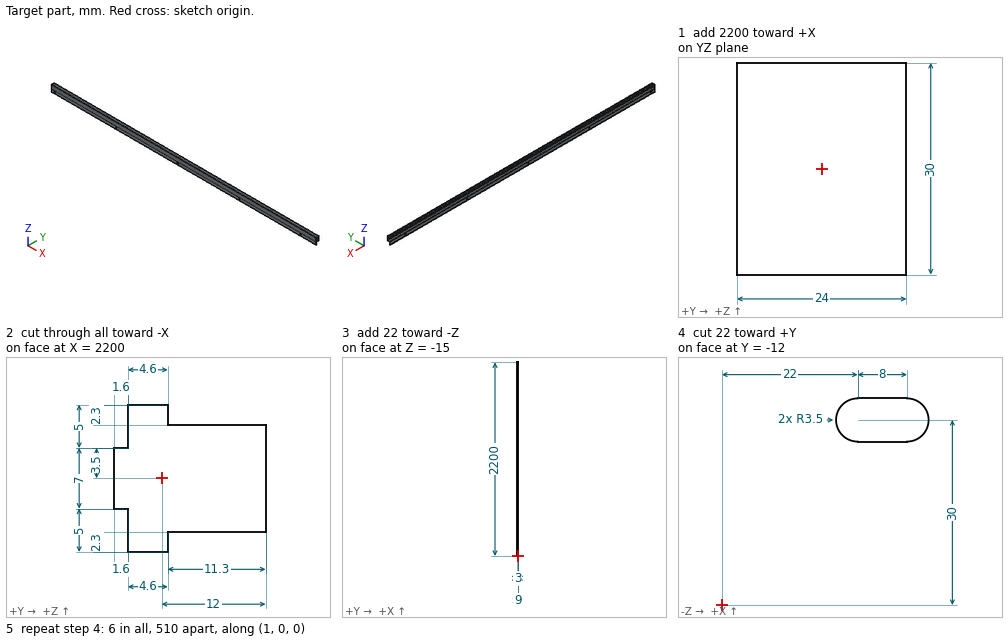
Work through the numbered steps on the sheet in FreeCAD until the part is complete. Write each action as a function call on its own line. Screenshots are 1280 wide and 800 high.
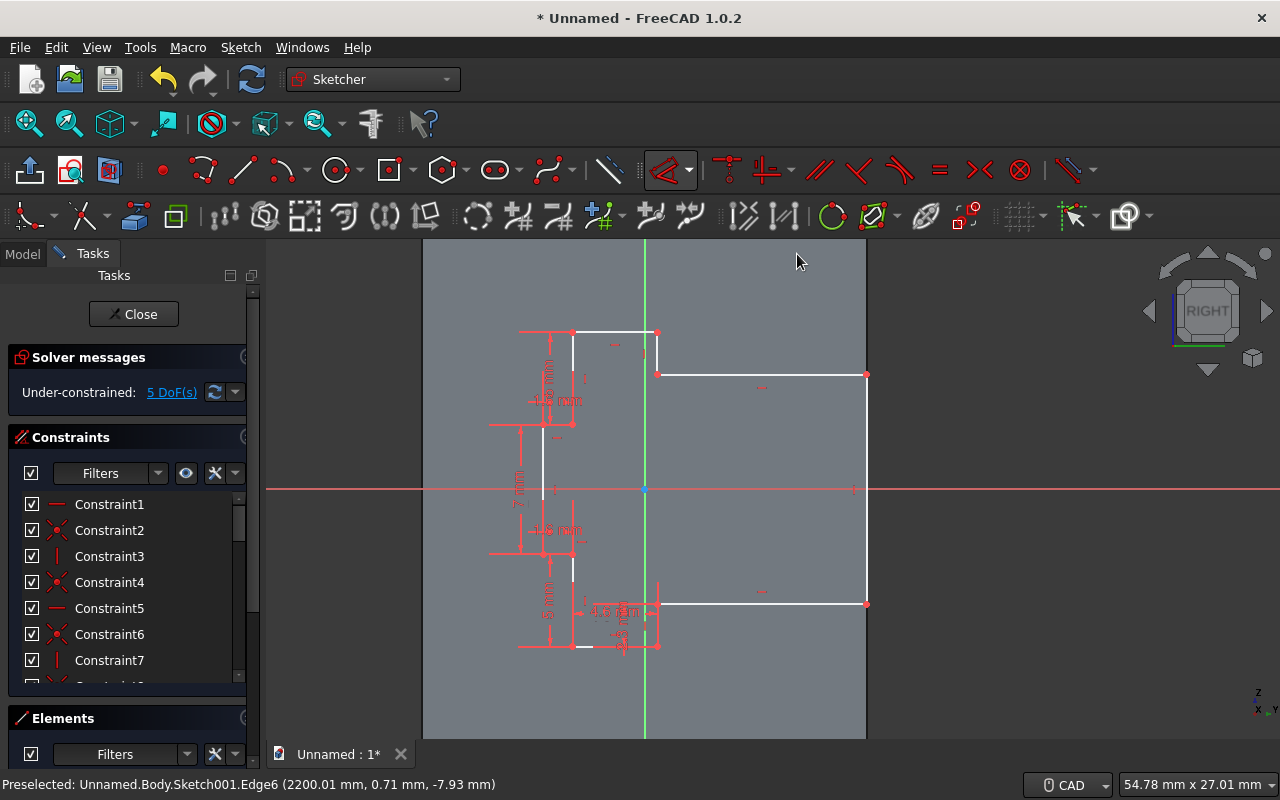
click(657, 362)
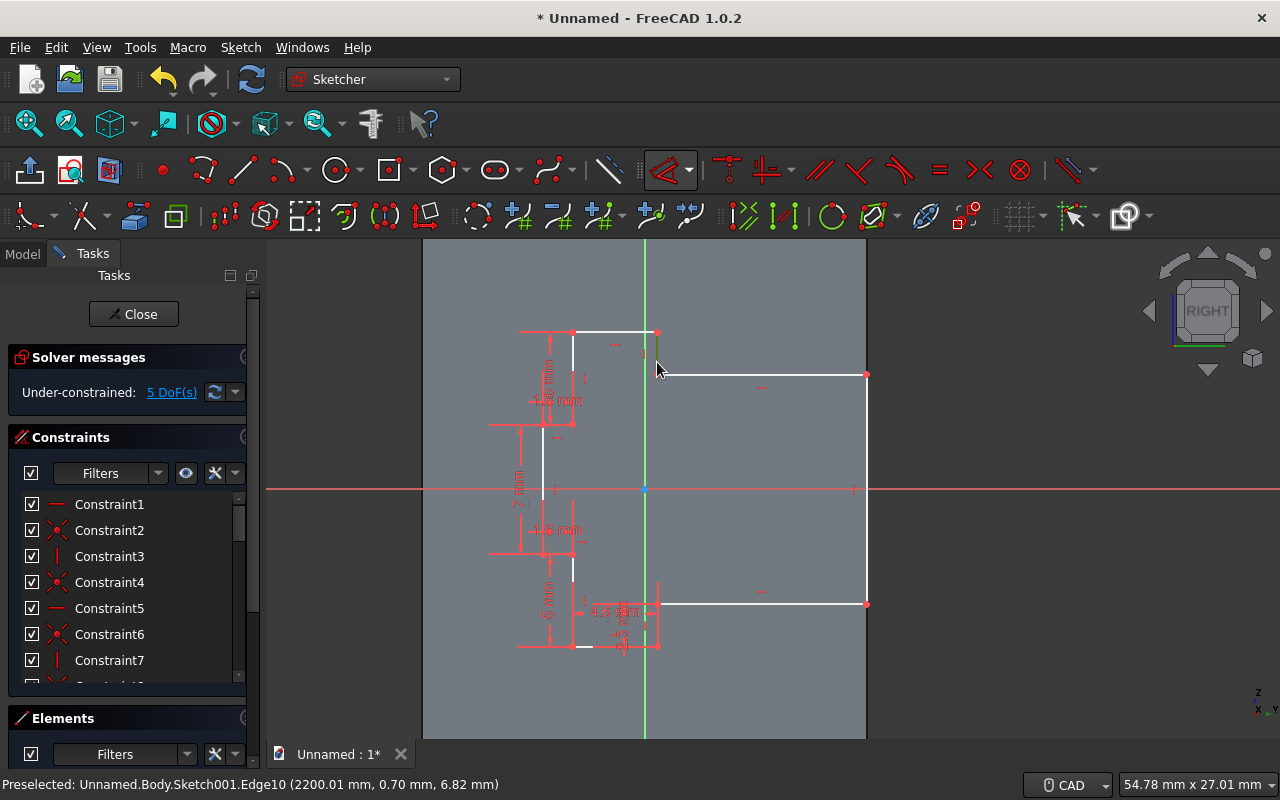
key(i)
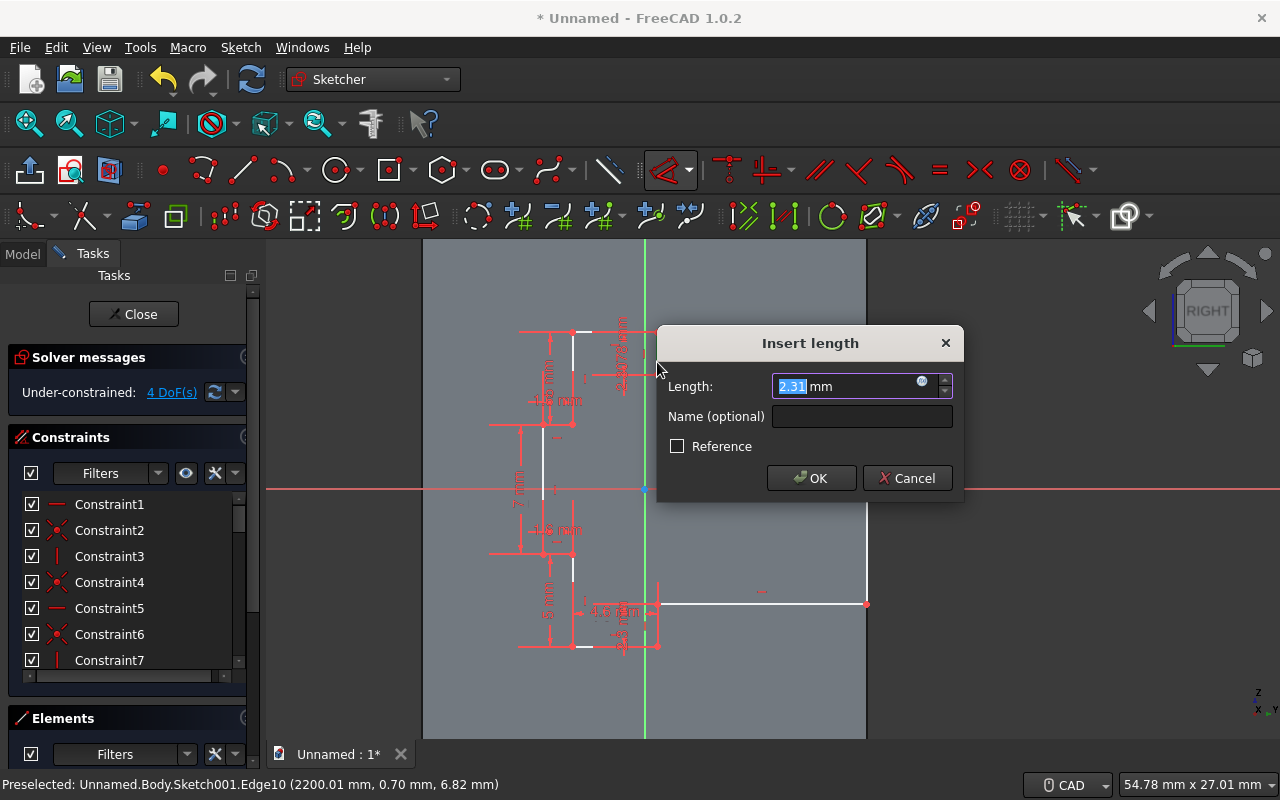
text(2.3)
key(Return)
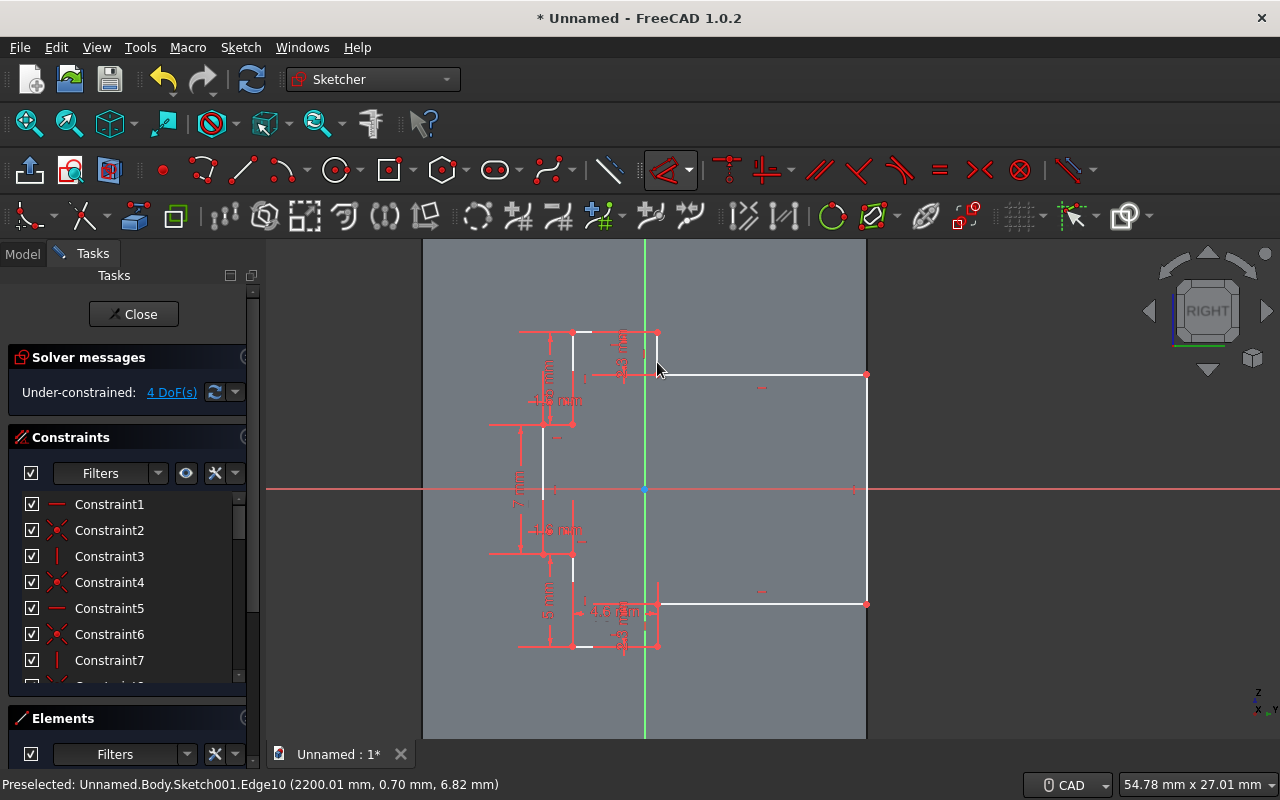
click(598, 332)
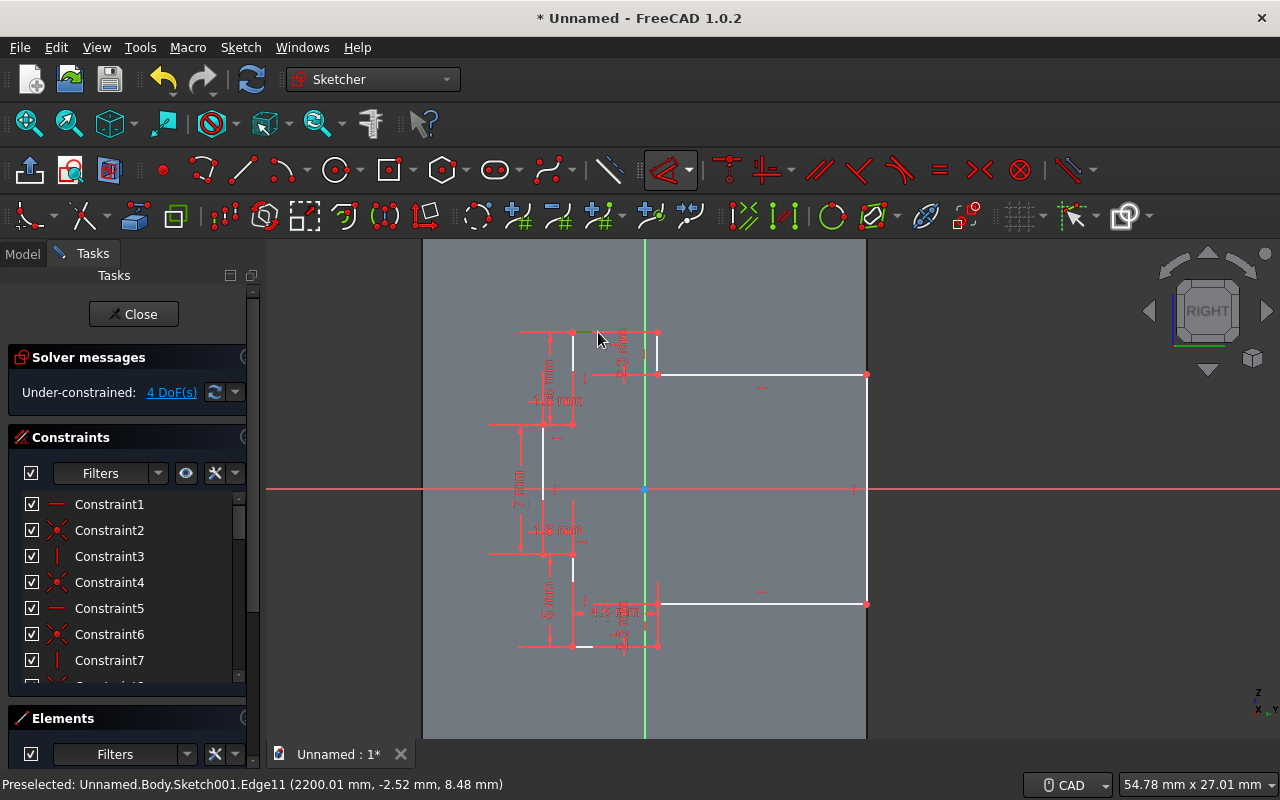
click(692, 170)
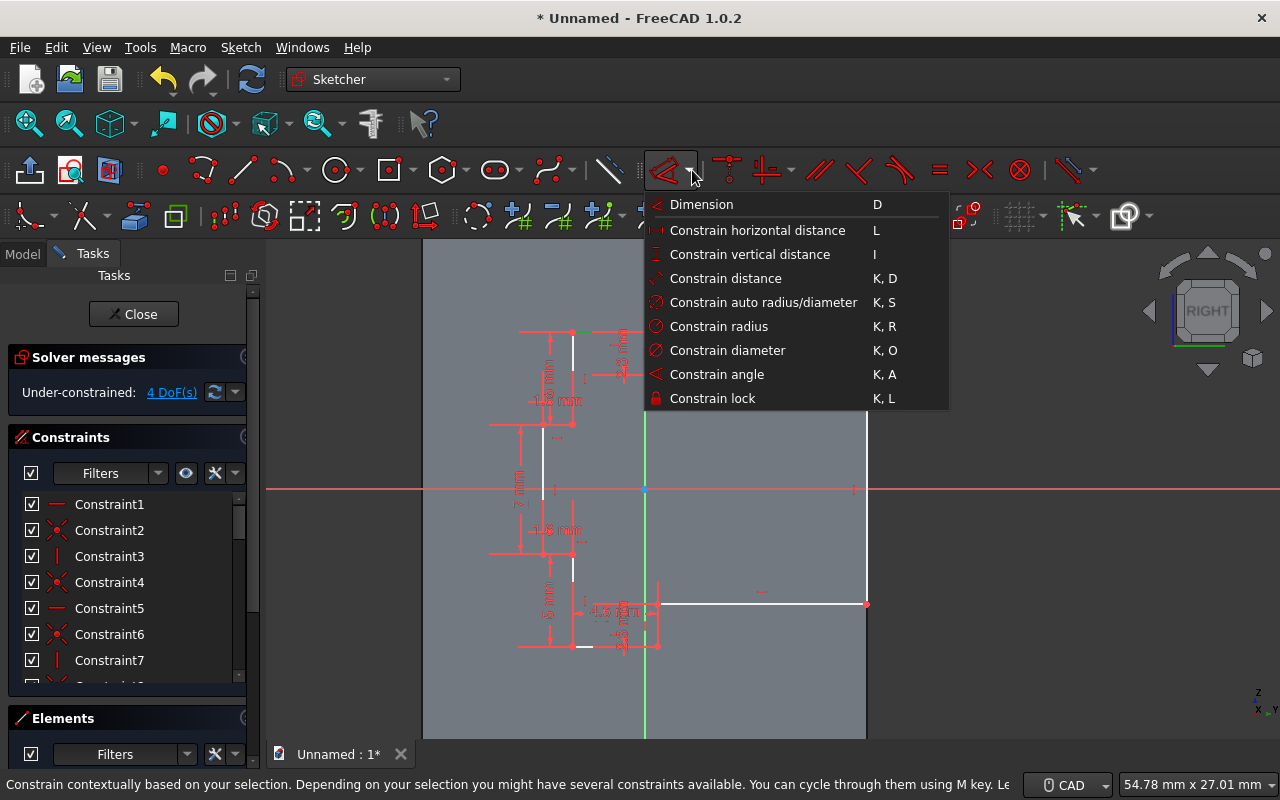
click(797, 230)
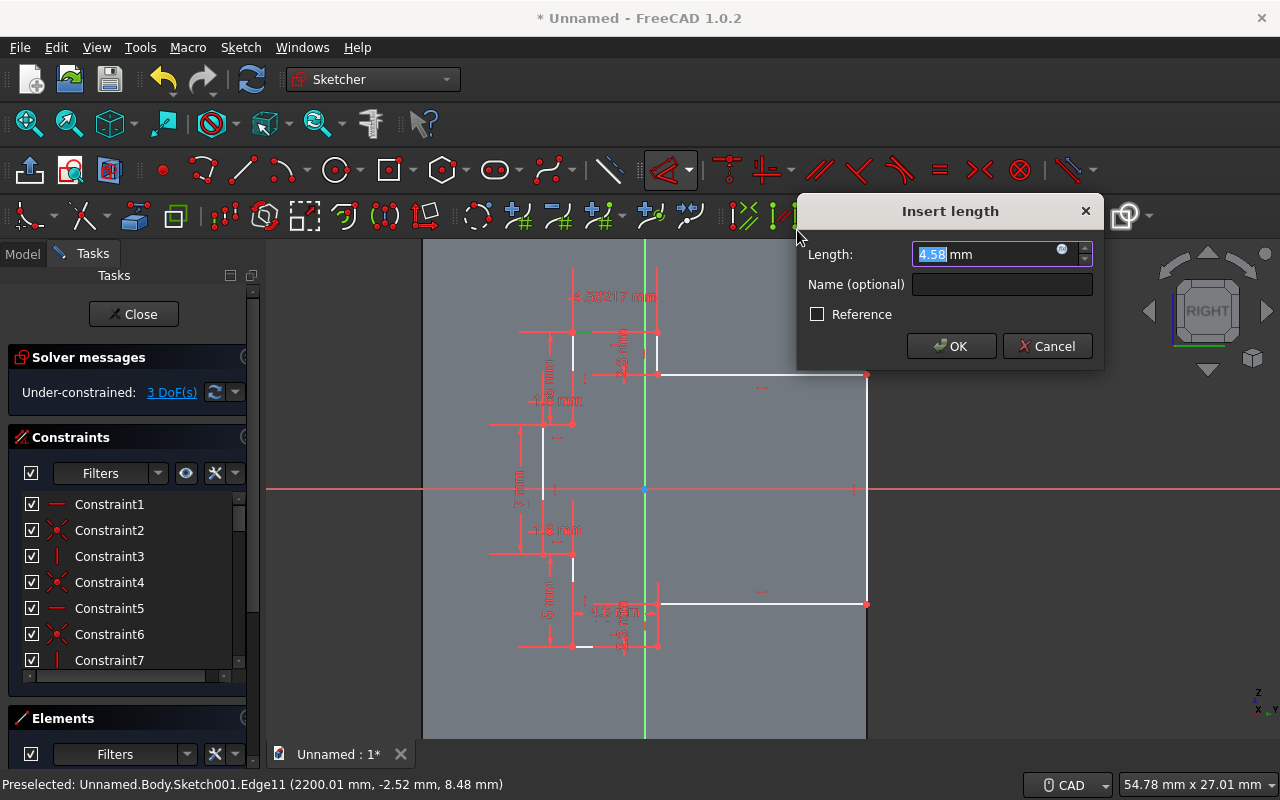
text(4.6)
key(Return)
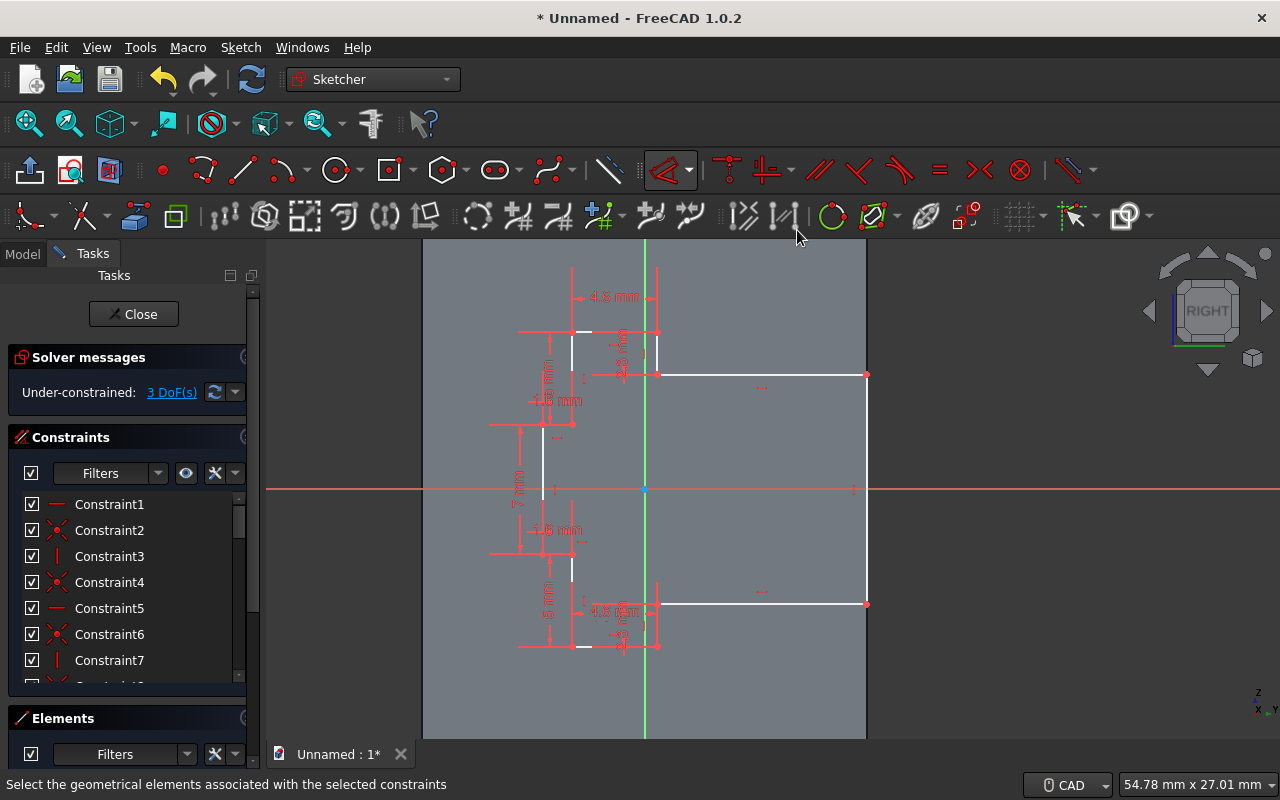
click(867, 604)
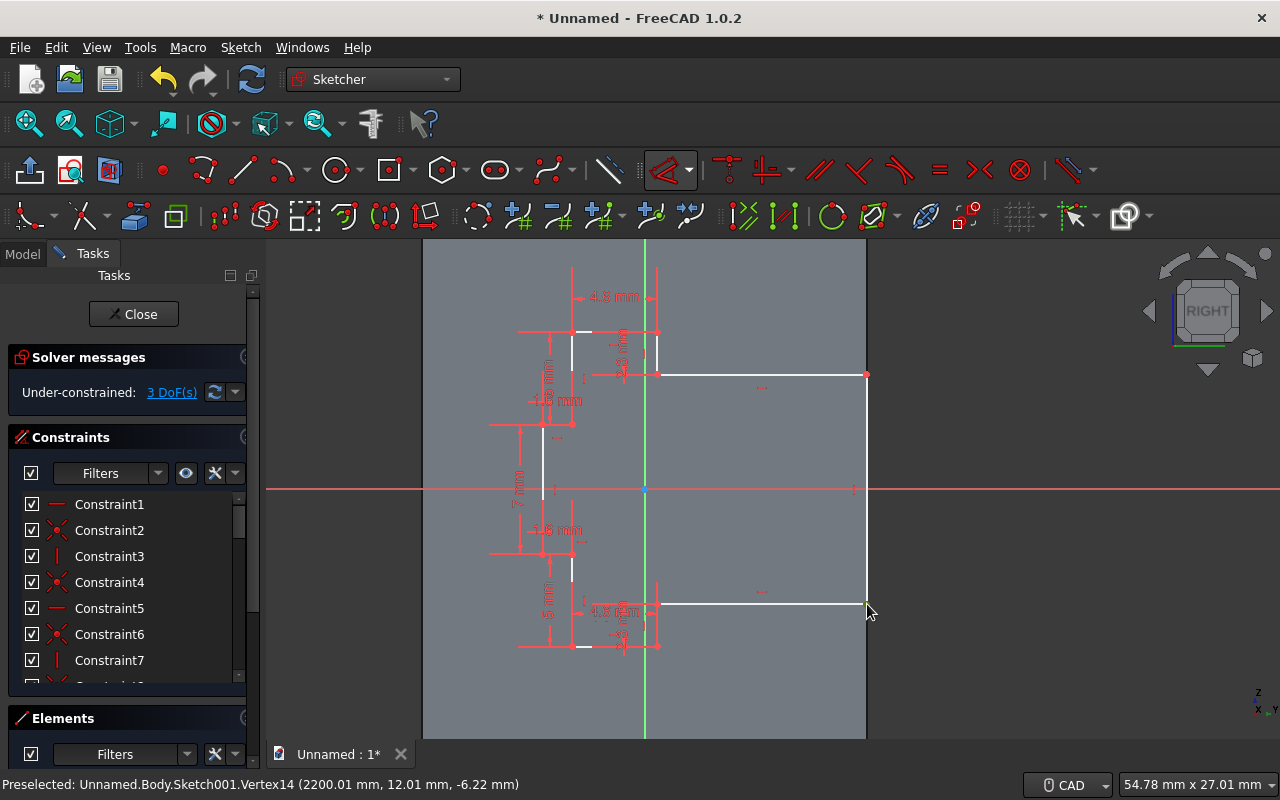
key(l)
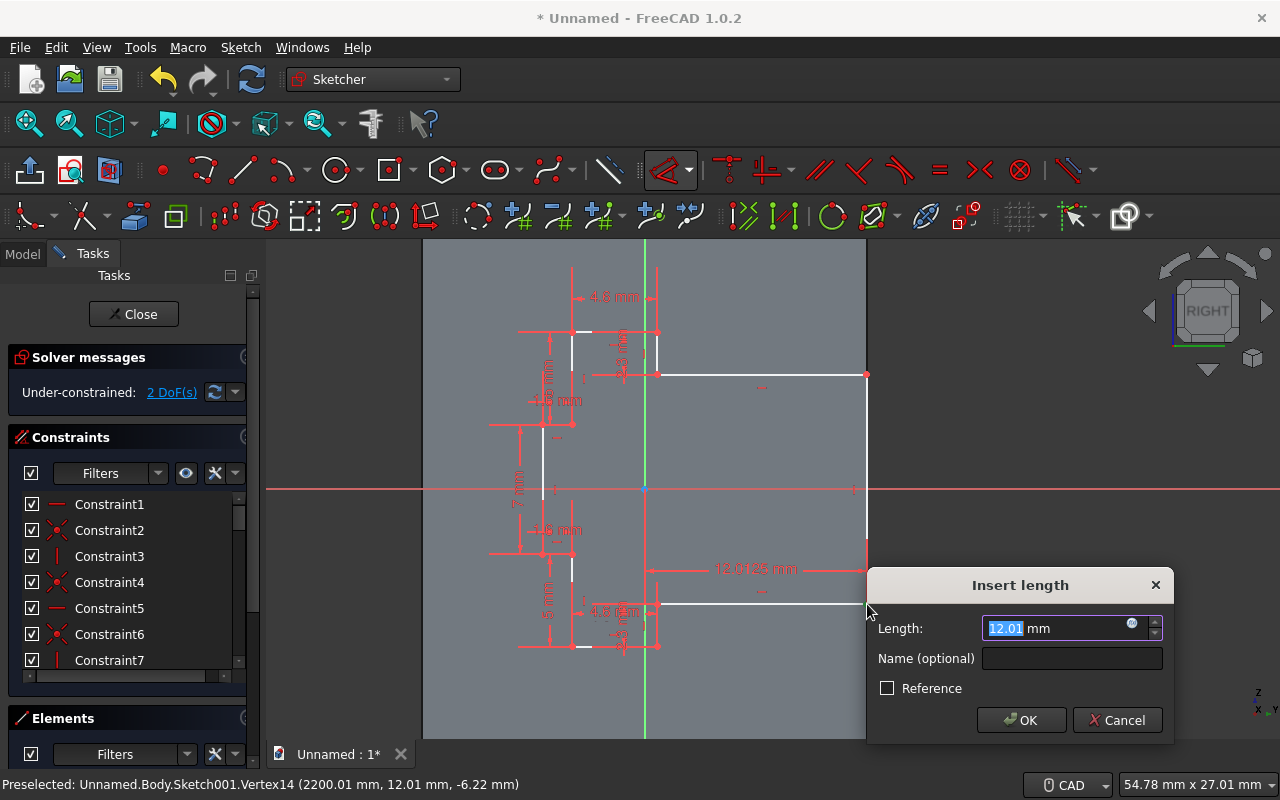
text(12)
key(Return)